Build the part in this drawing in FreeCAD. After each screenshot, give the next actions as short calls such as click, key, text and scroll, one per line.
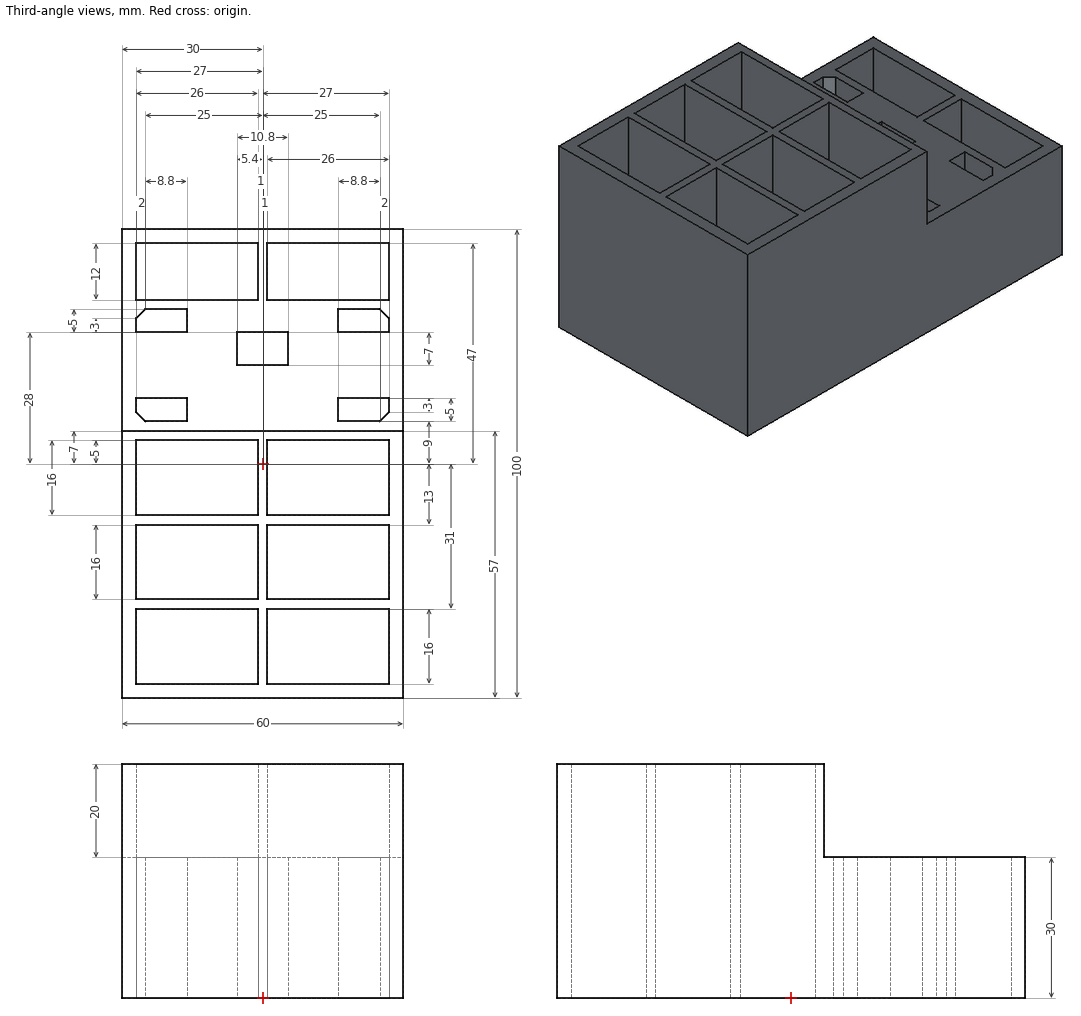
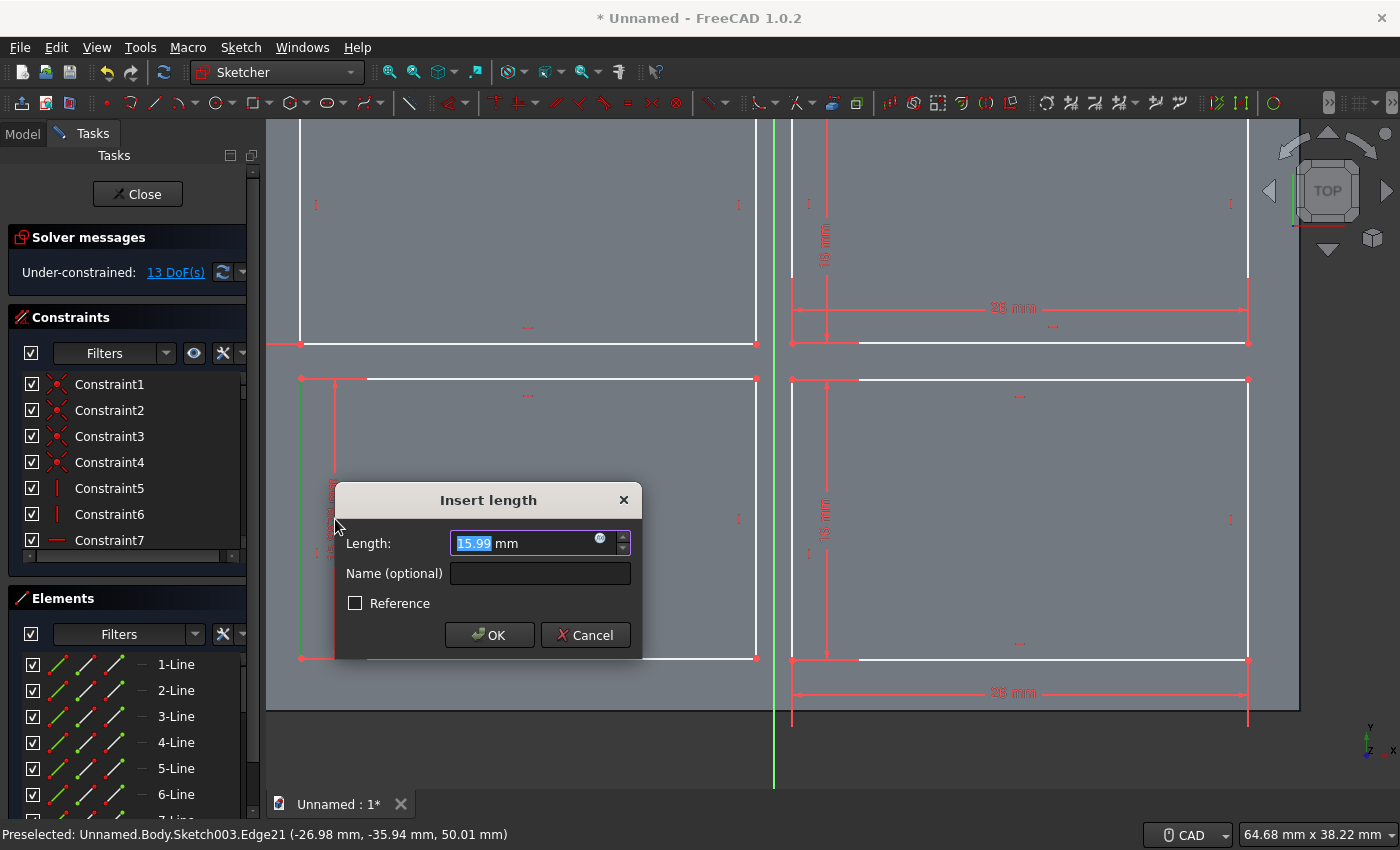
text(16)
key(Return)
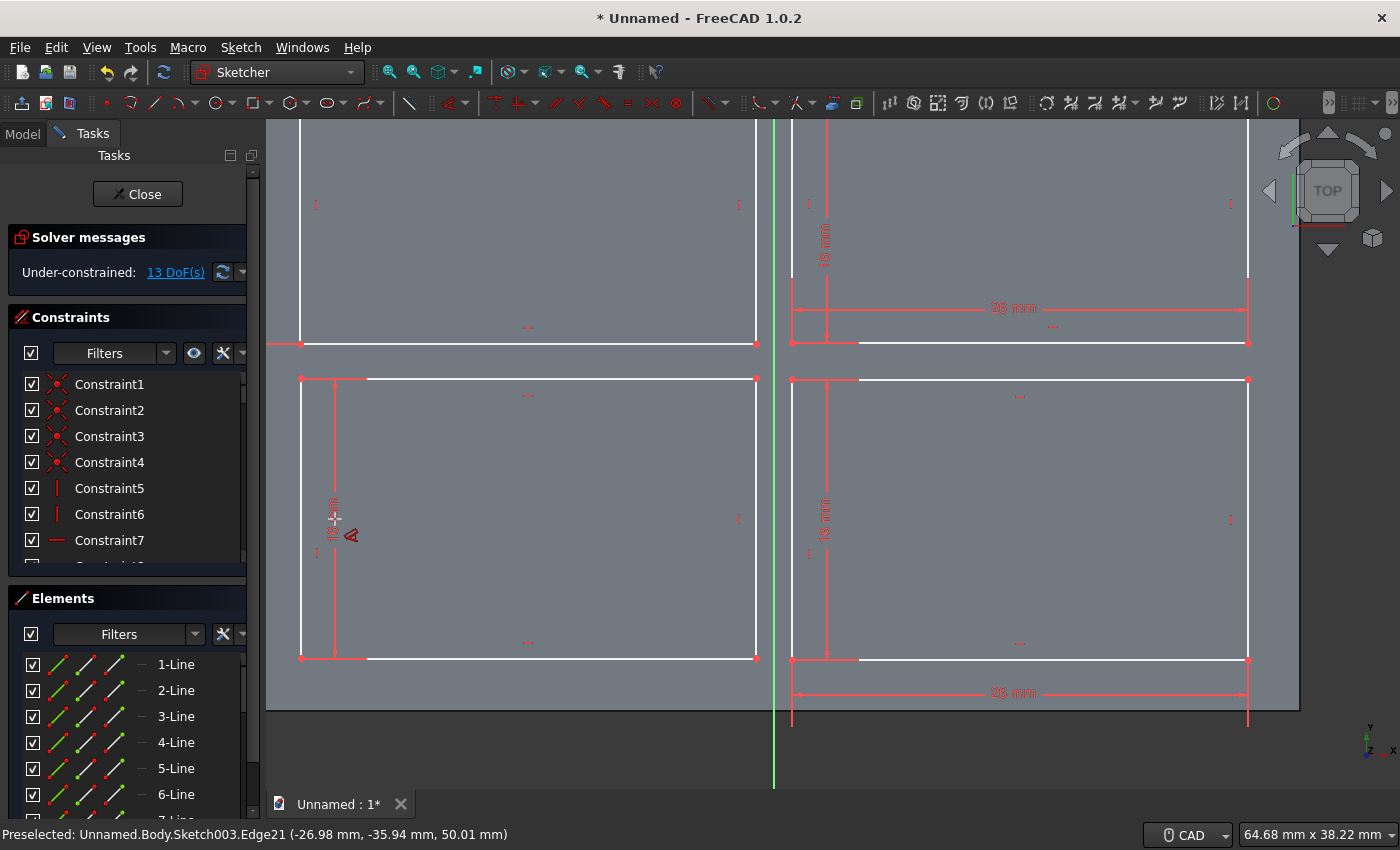
click(438, 659)
click(529, 693)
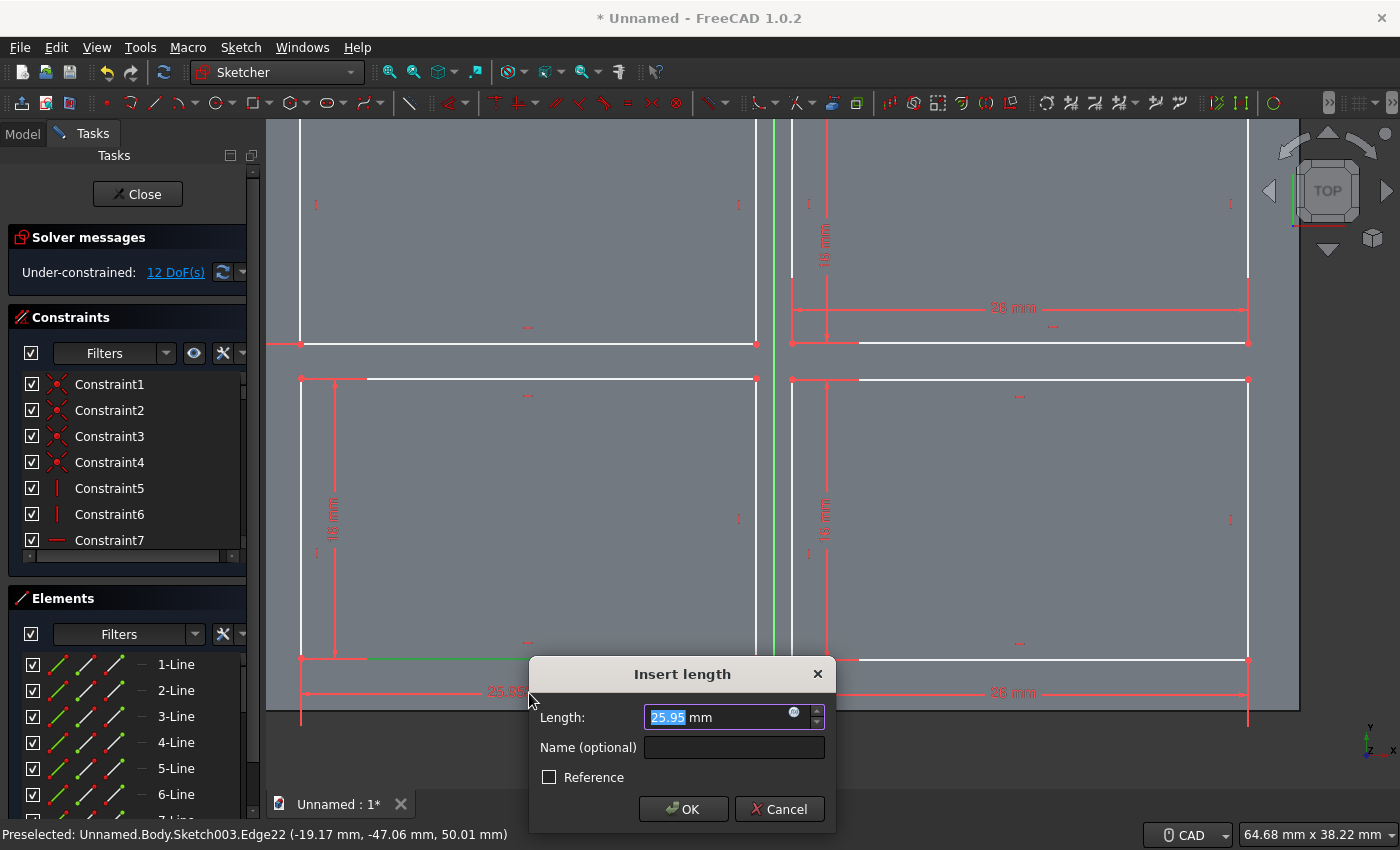
text(26)
key(Return)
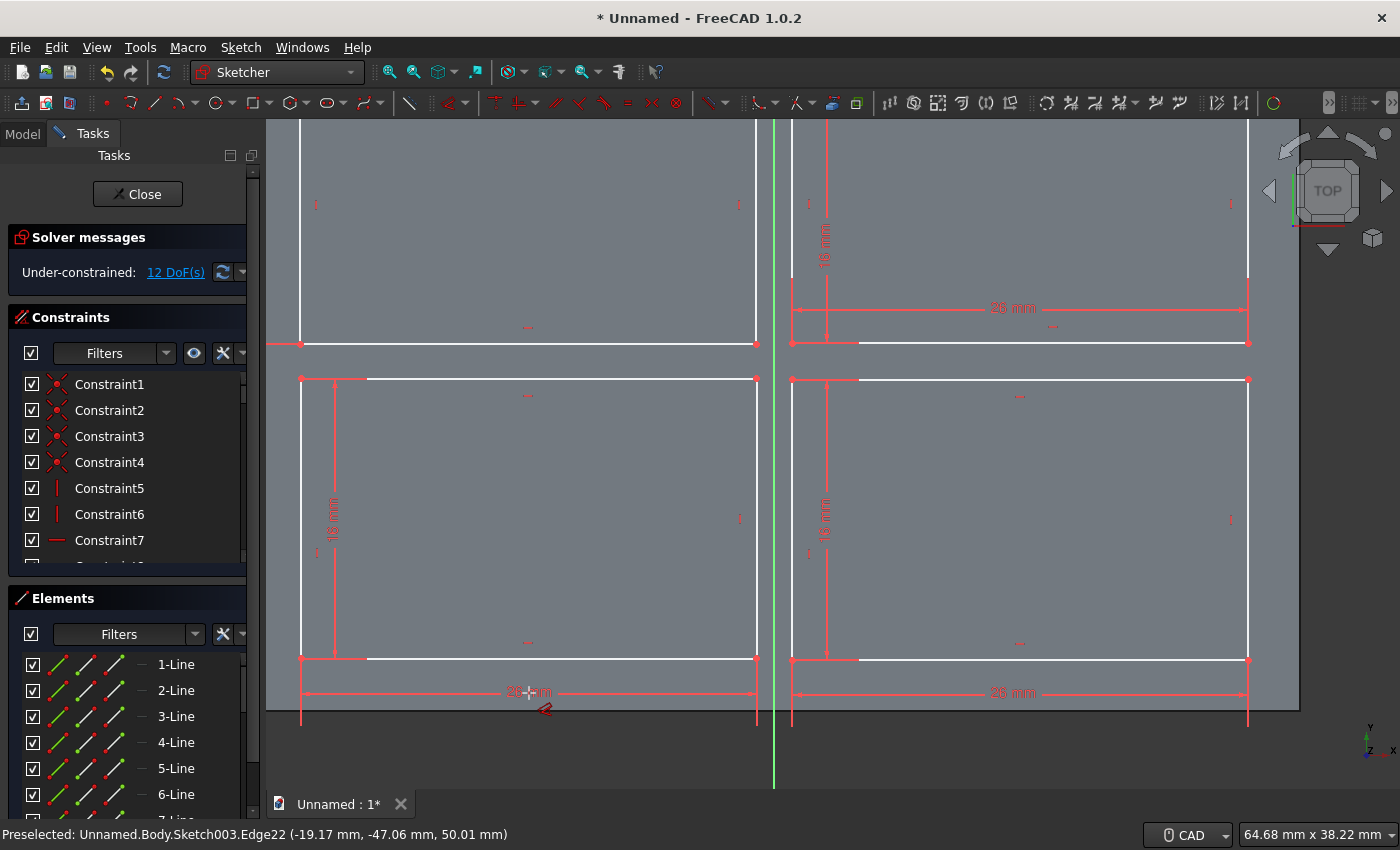
scroll(757, 659, down, 4)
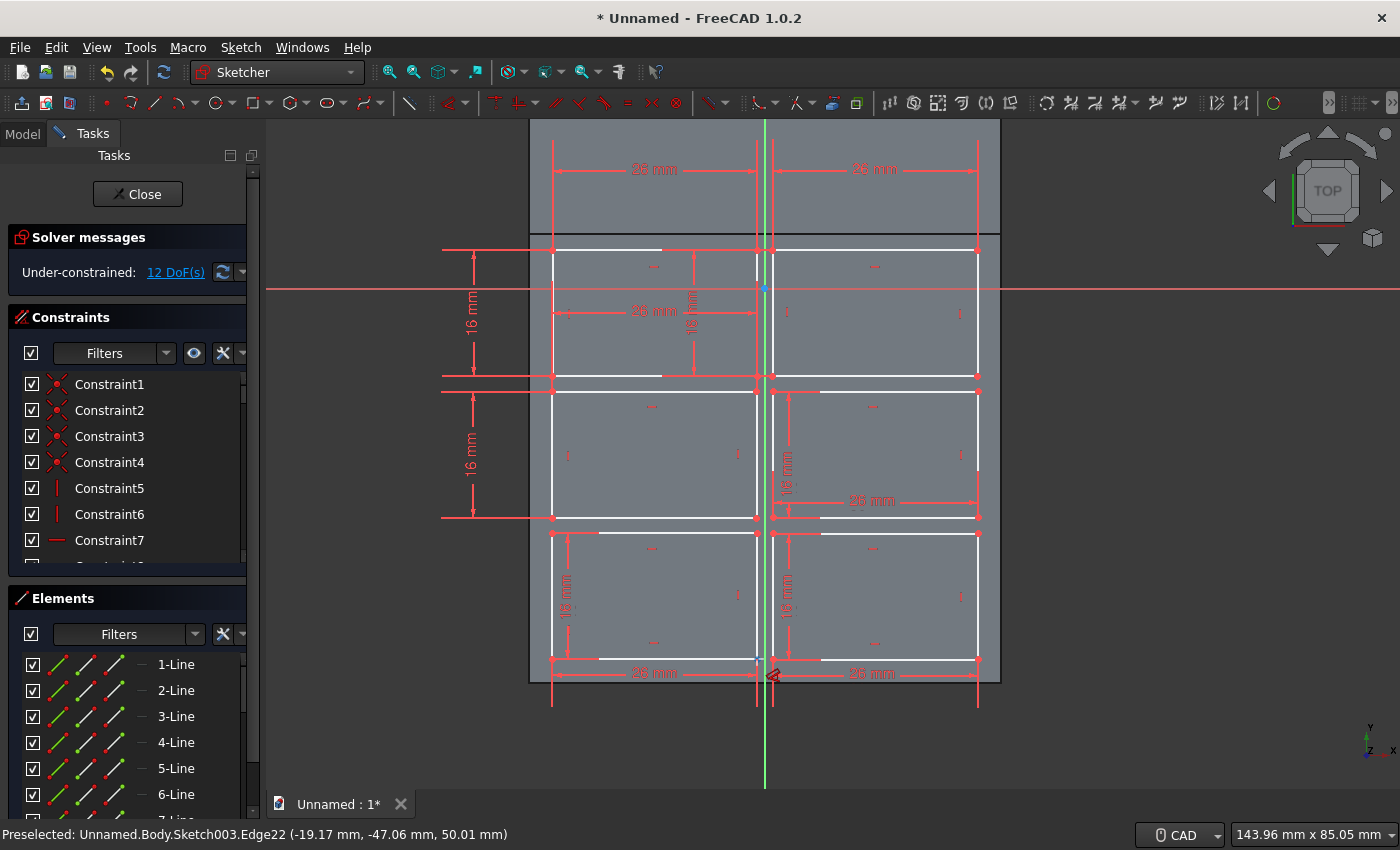
click(553, 250)
click(519, 269)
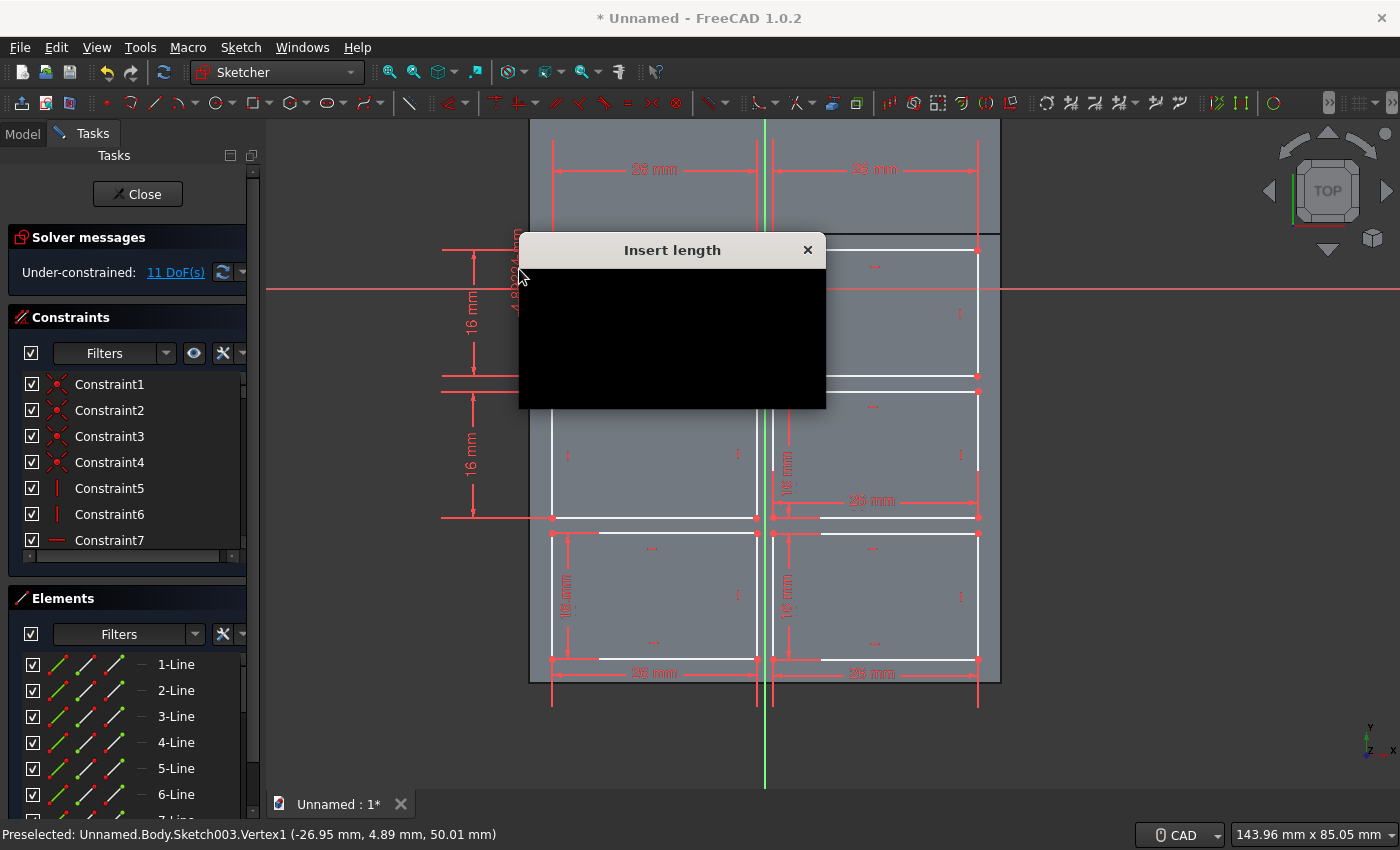
text(5)
key(Return)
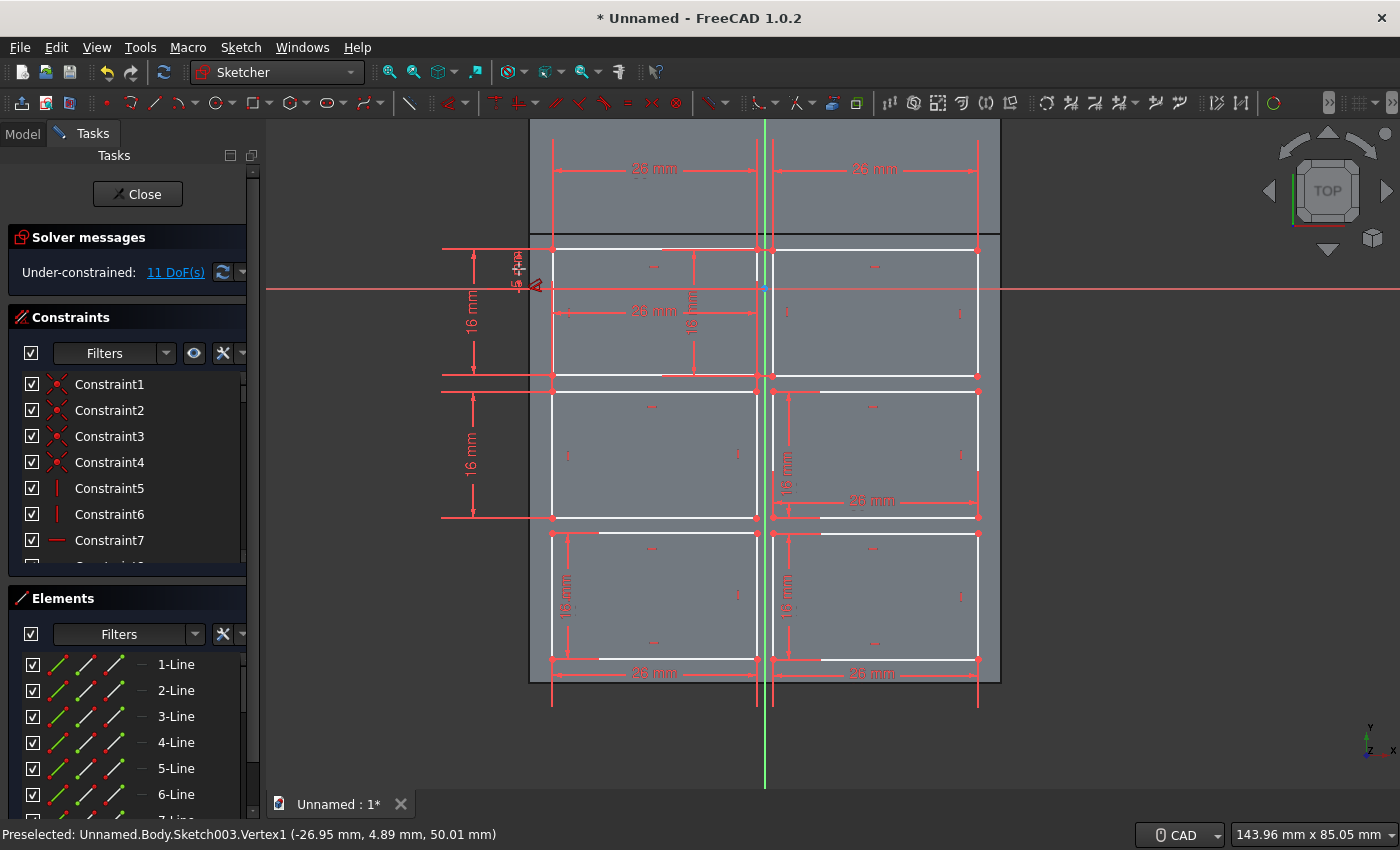
scroll(757, 375, up, 9)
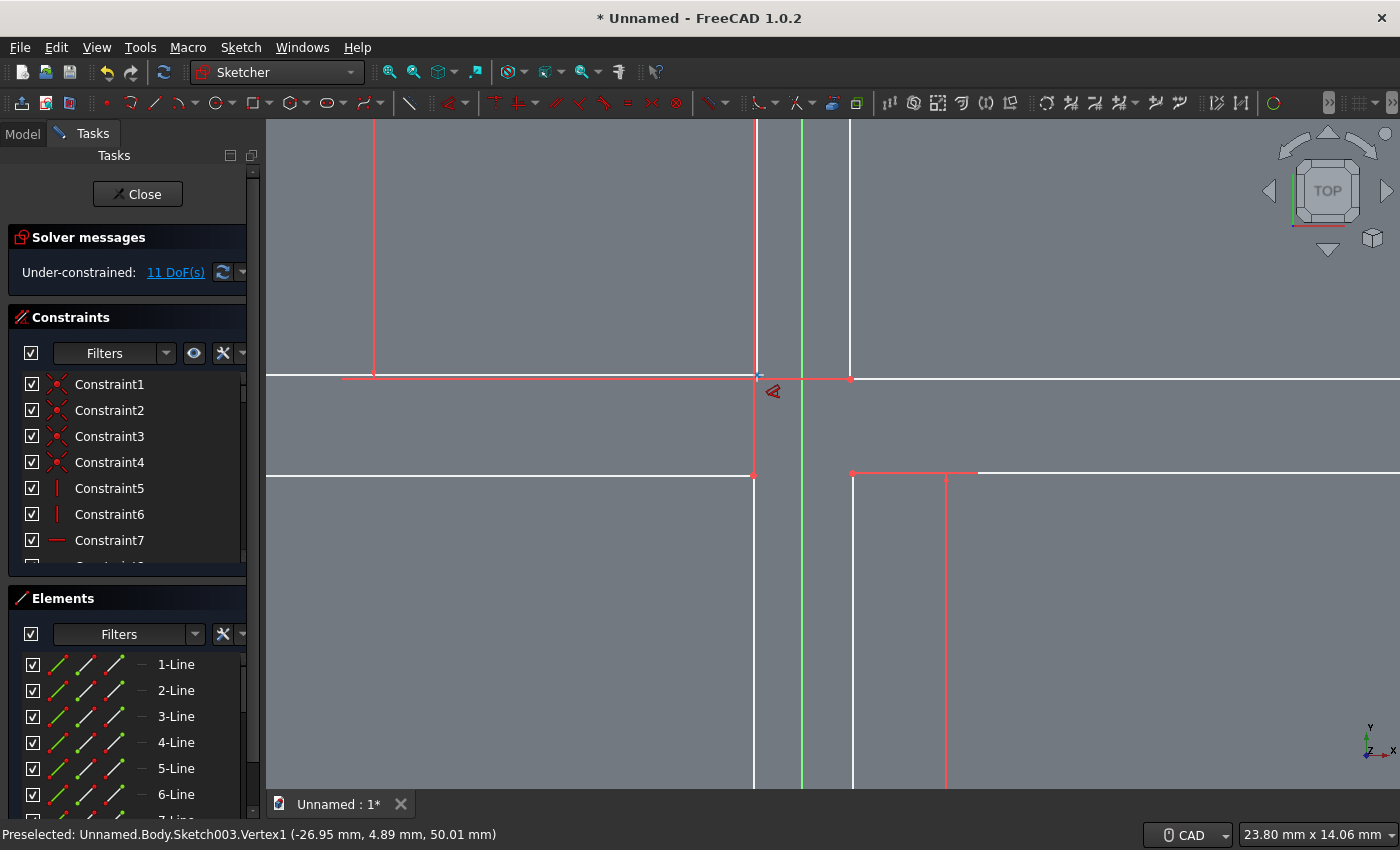
click(757, 375)
click(780, 409)